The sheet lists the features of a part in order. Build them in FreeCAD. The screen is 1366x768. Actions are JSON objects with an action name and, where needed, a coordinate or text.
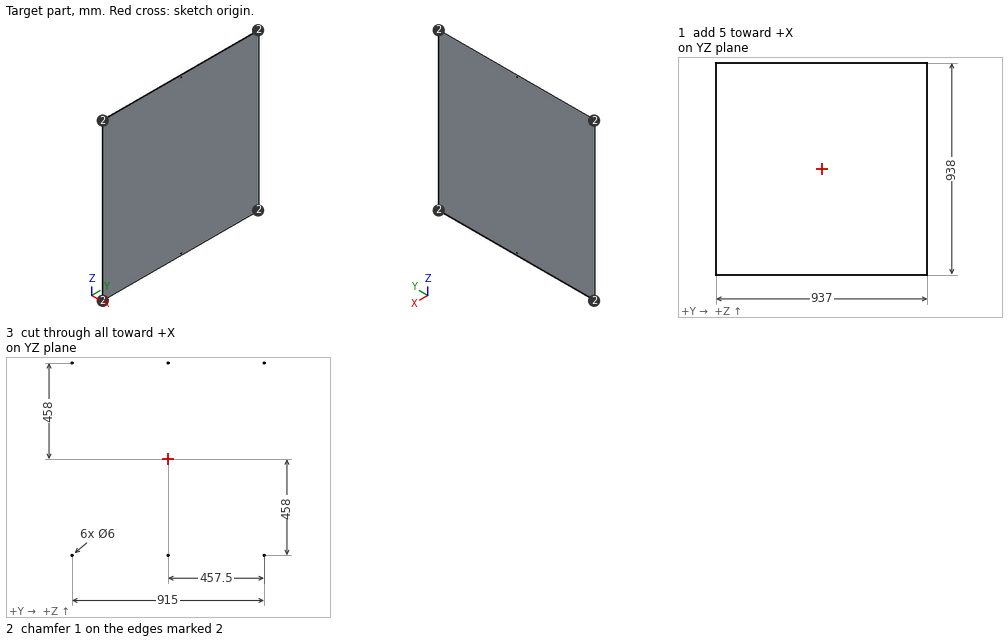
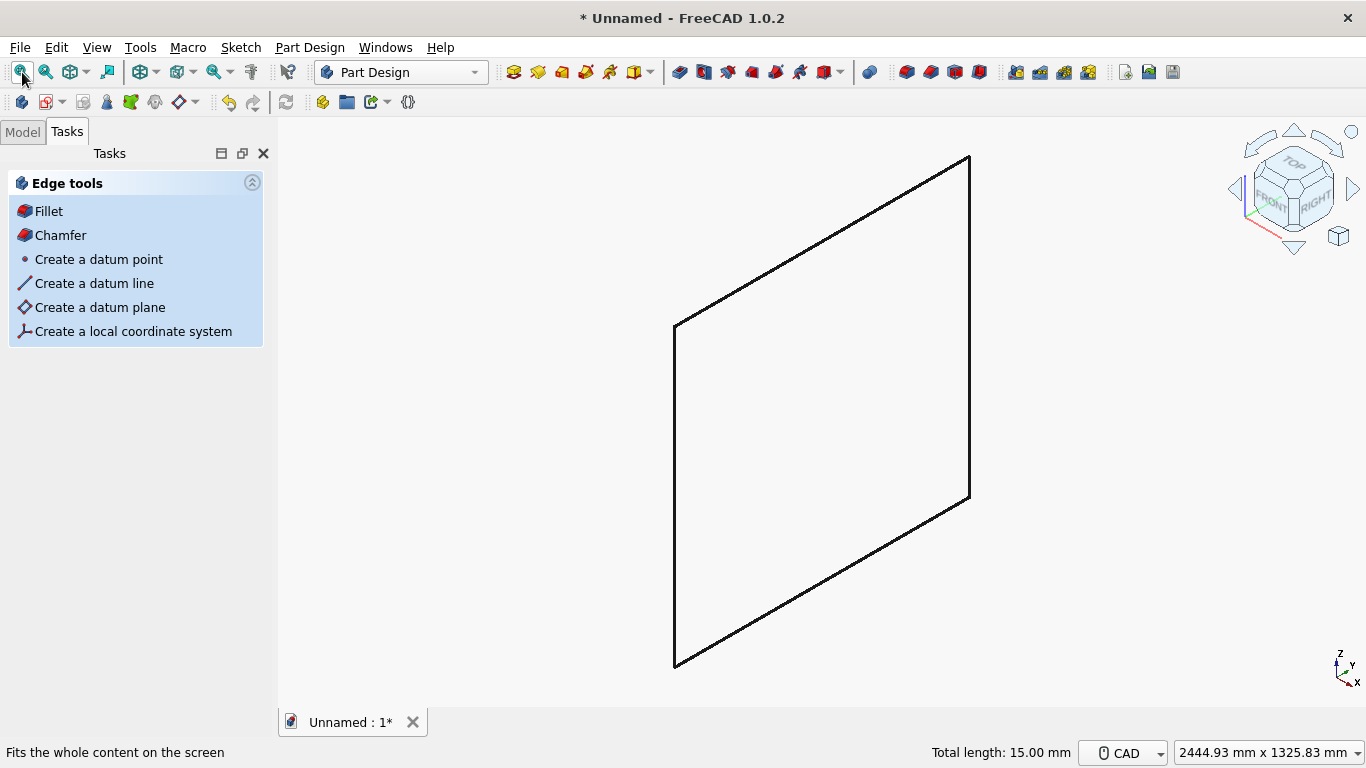
{"action": "scroll", "coordinate": [675, 326], "scroll_direction": "up", "scroll_amount": 15}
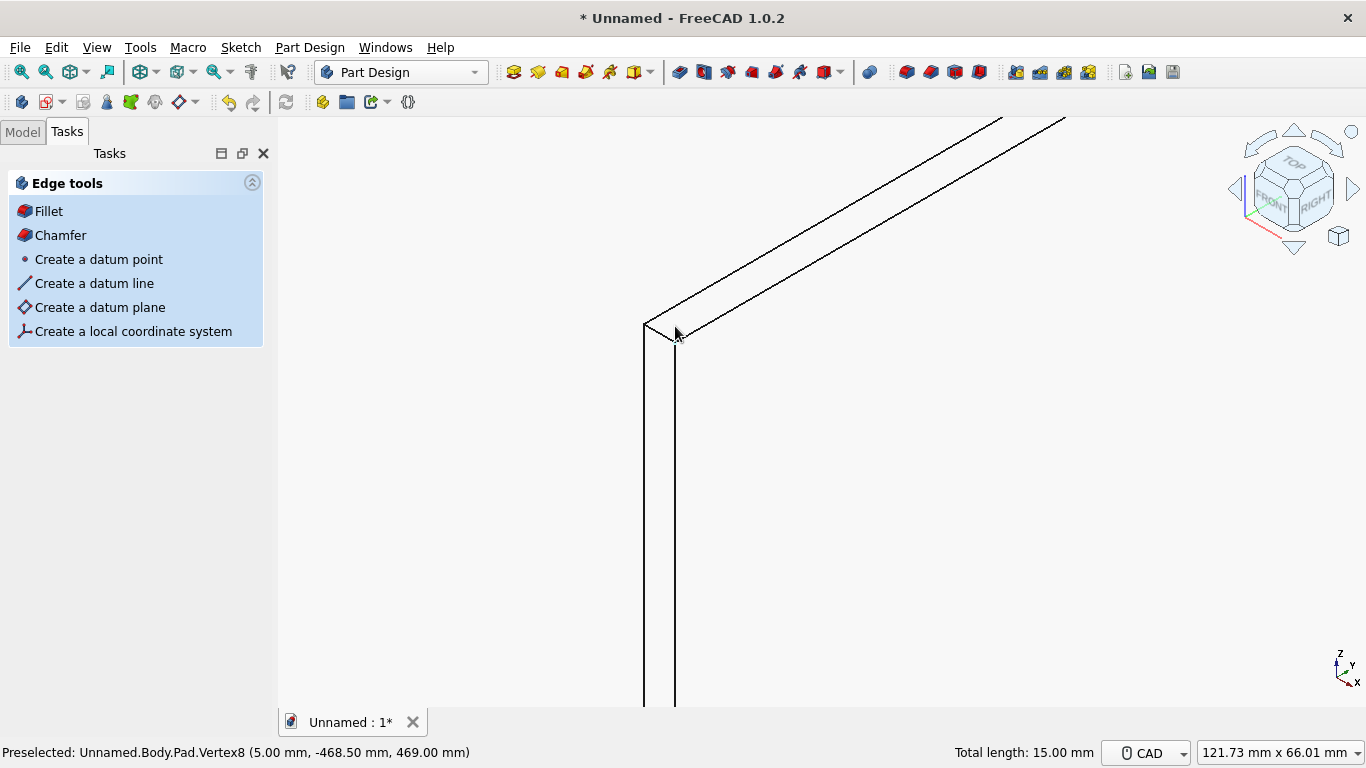
{"action": "left_click", "coordinate": [660, 332], "text": "ctrl"}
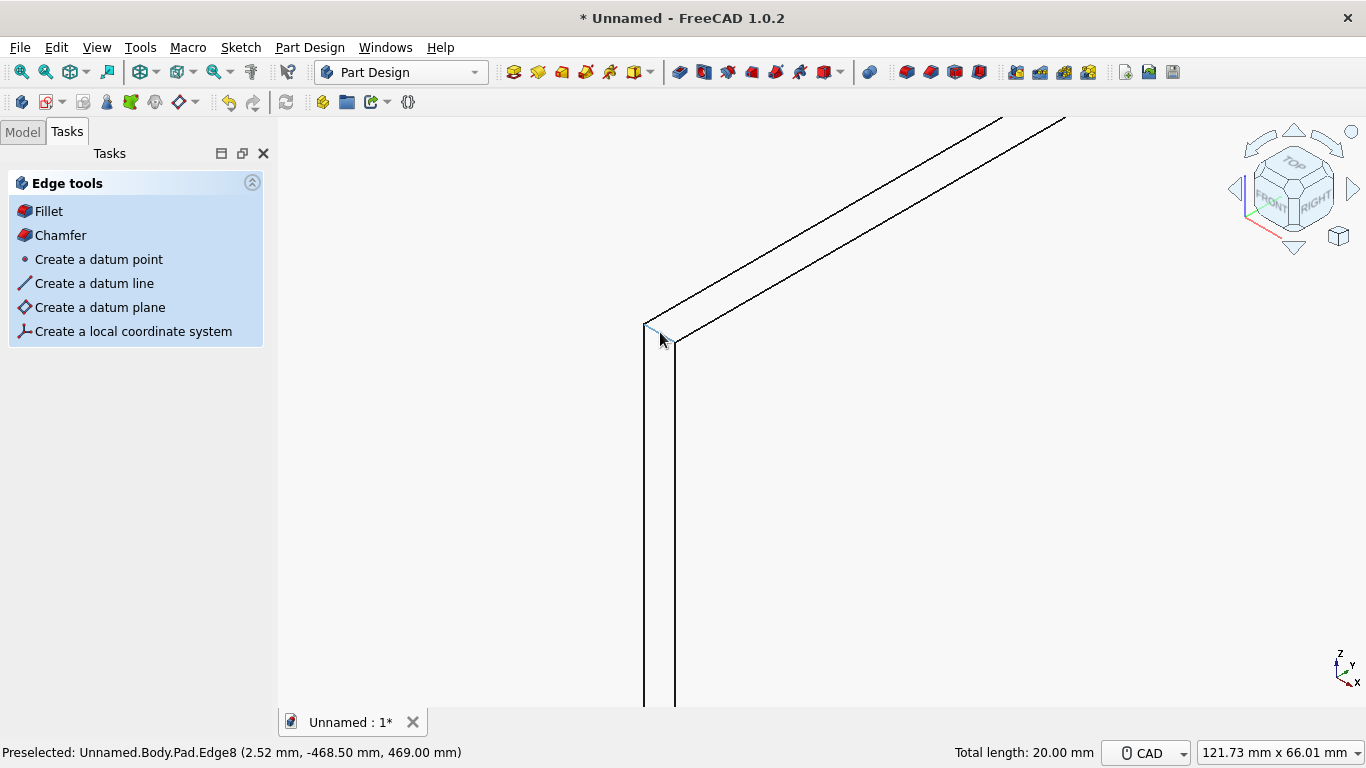
{"action": "key", "text": "v 1"}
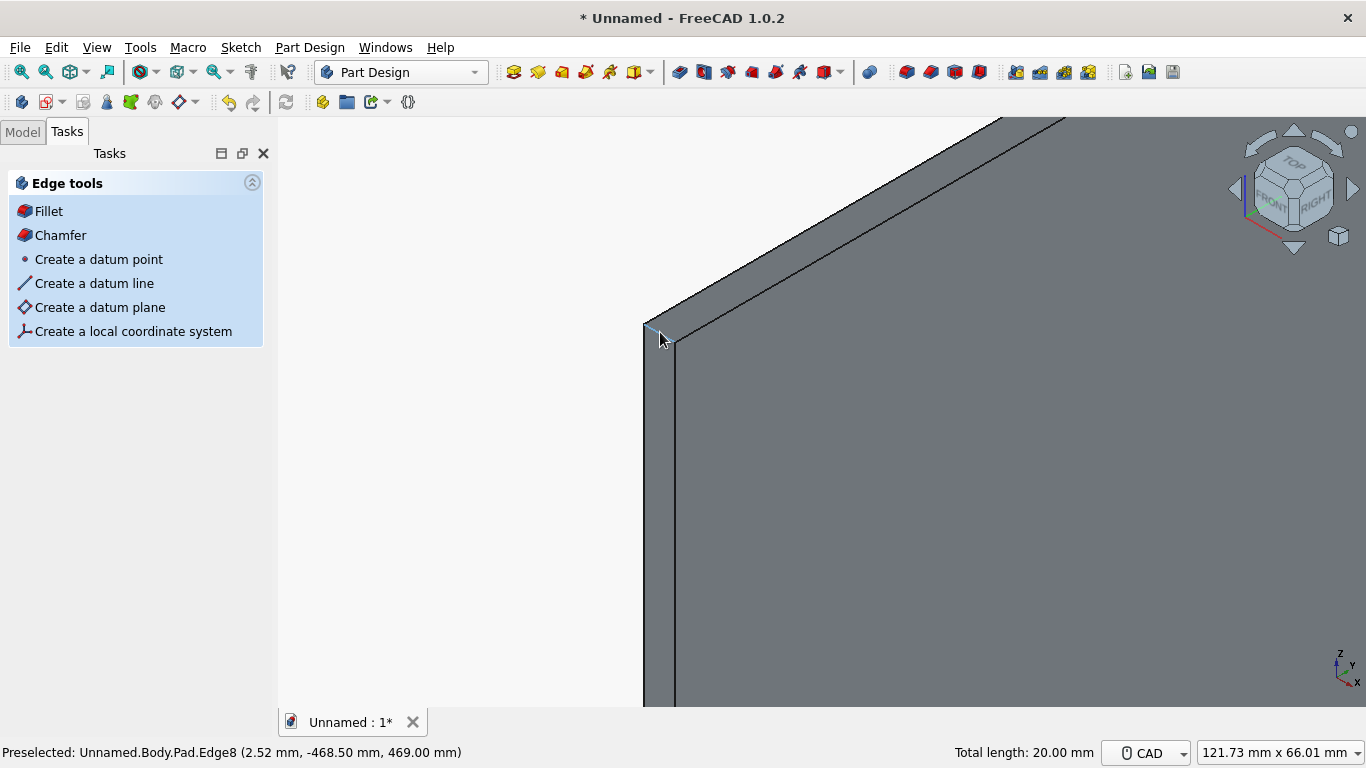
{"action": "left_click", "coordinate": [932, 72]}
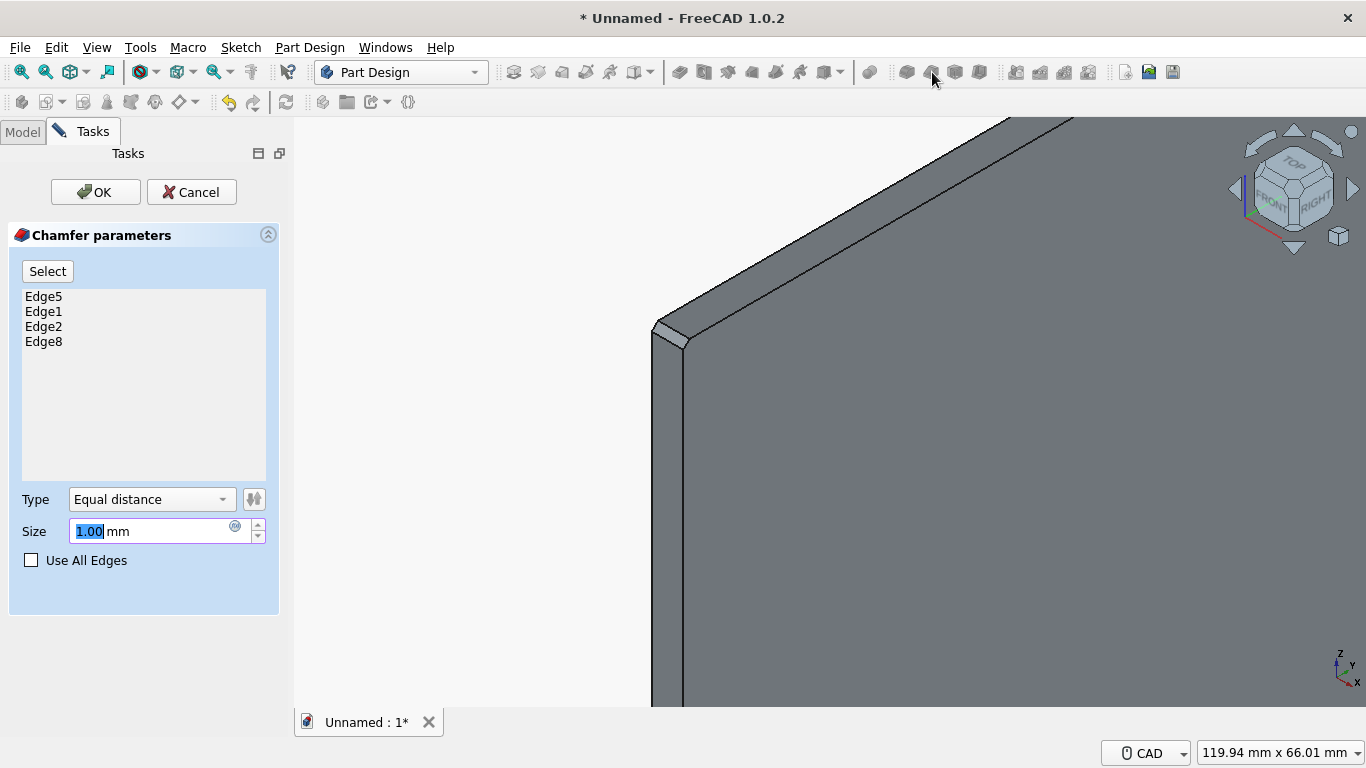
{"action": "type", "text": "1"}
{"action": "key", "text": "Tab"}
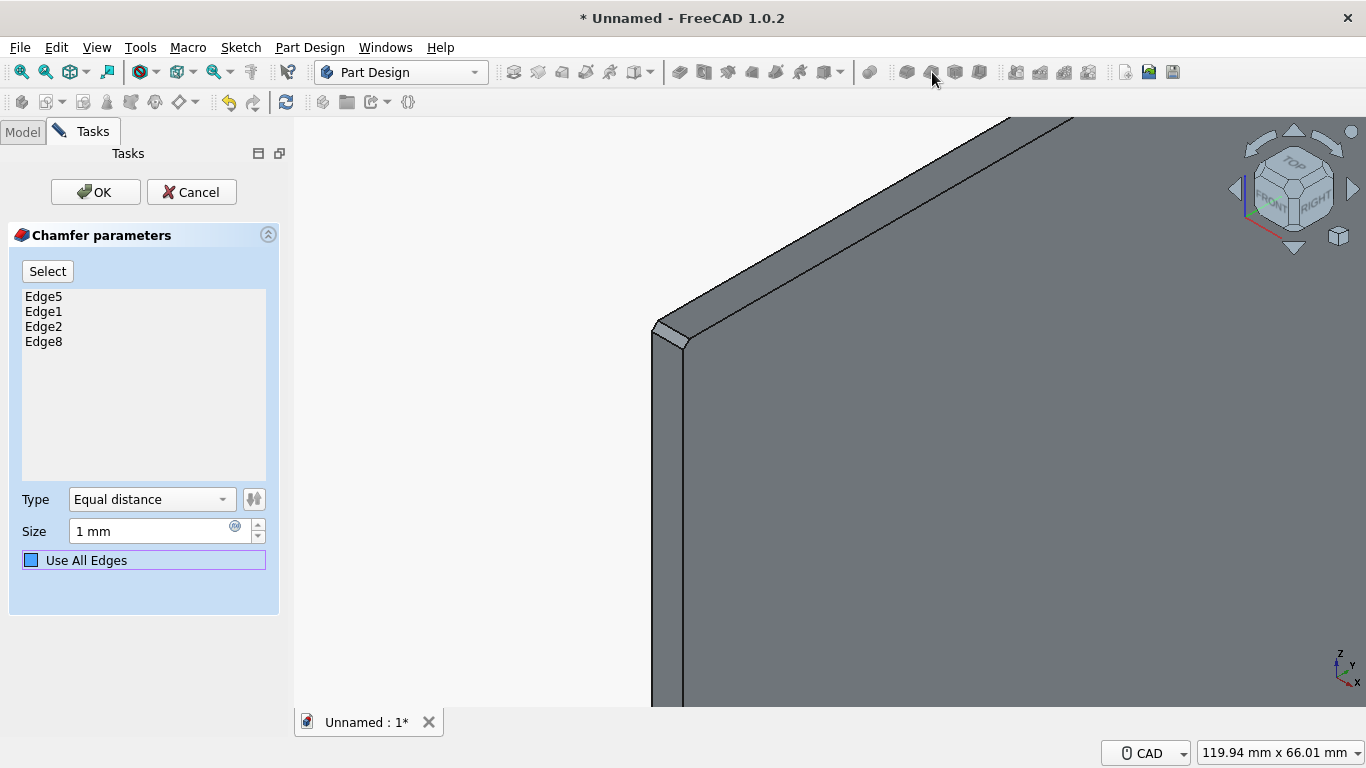
{"action": "left_click", "coordinate": [96, 192]}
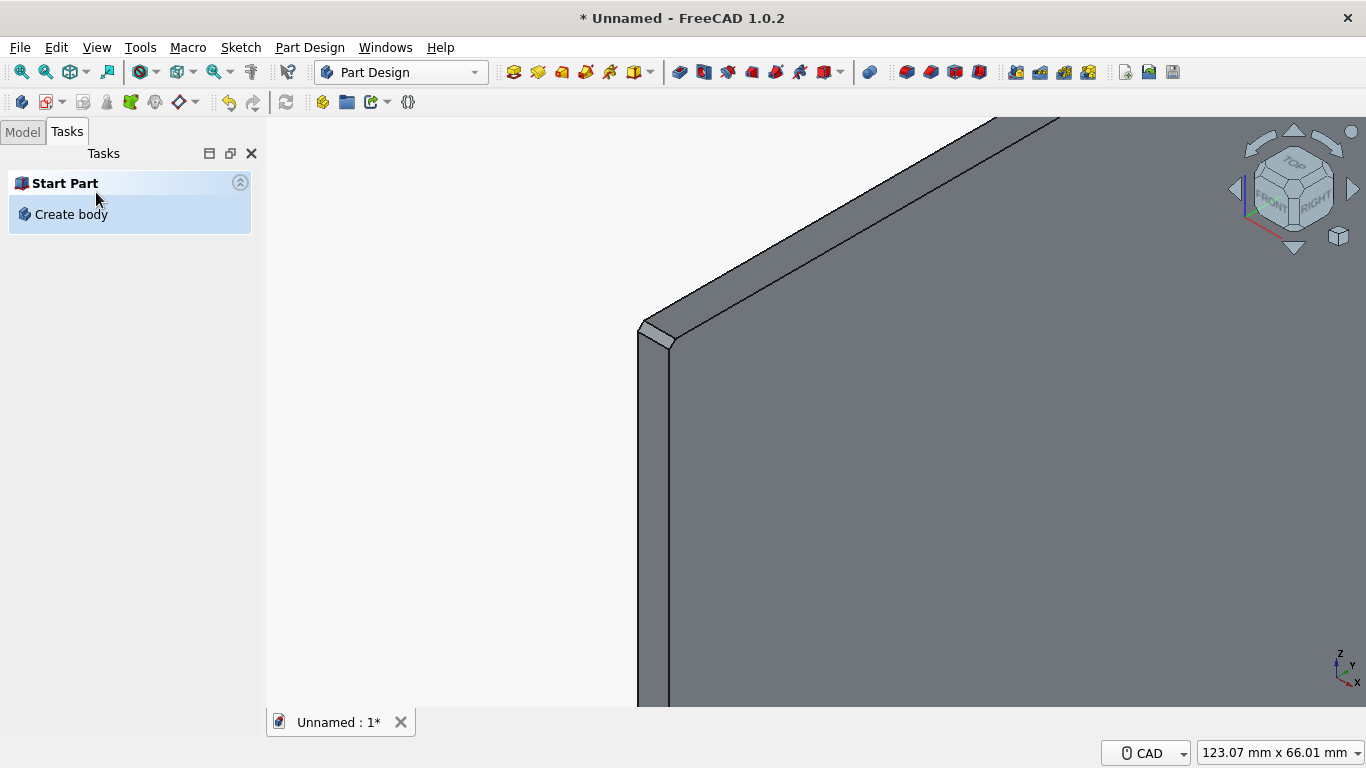
{"action": "left_click", "coordinate": [22, 72]}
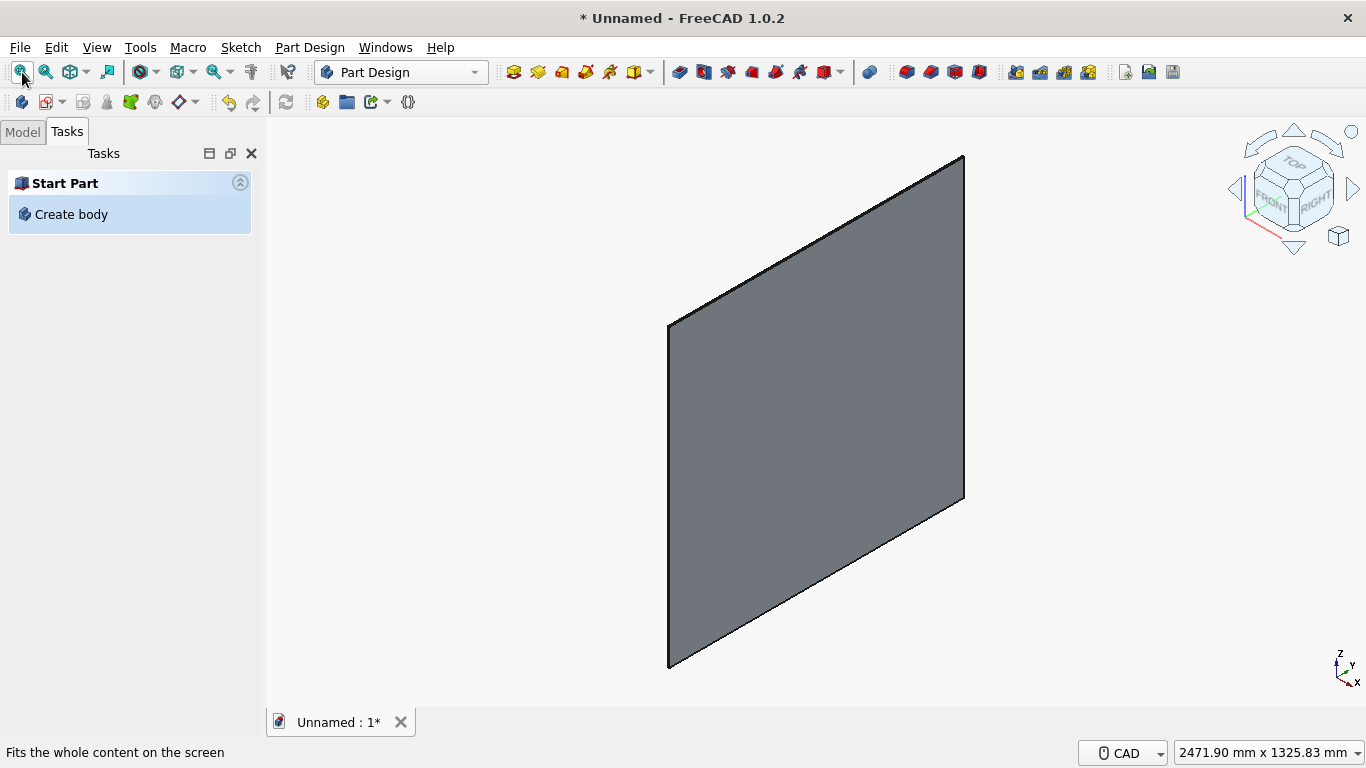
{"action": "left_click", "coordinate": [46, 102]}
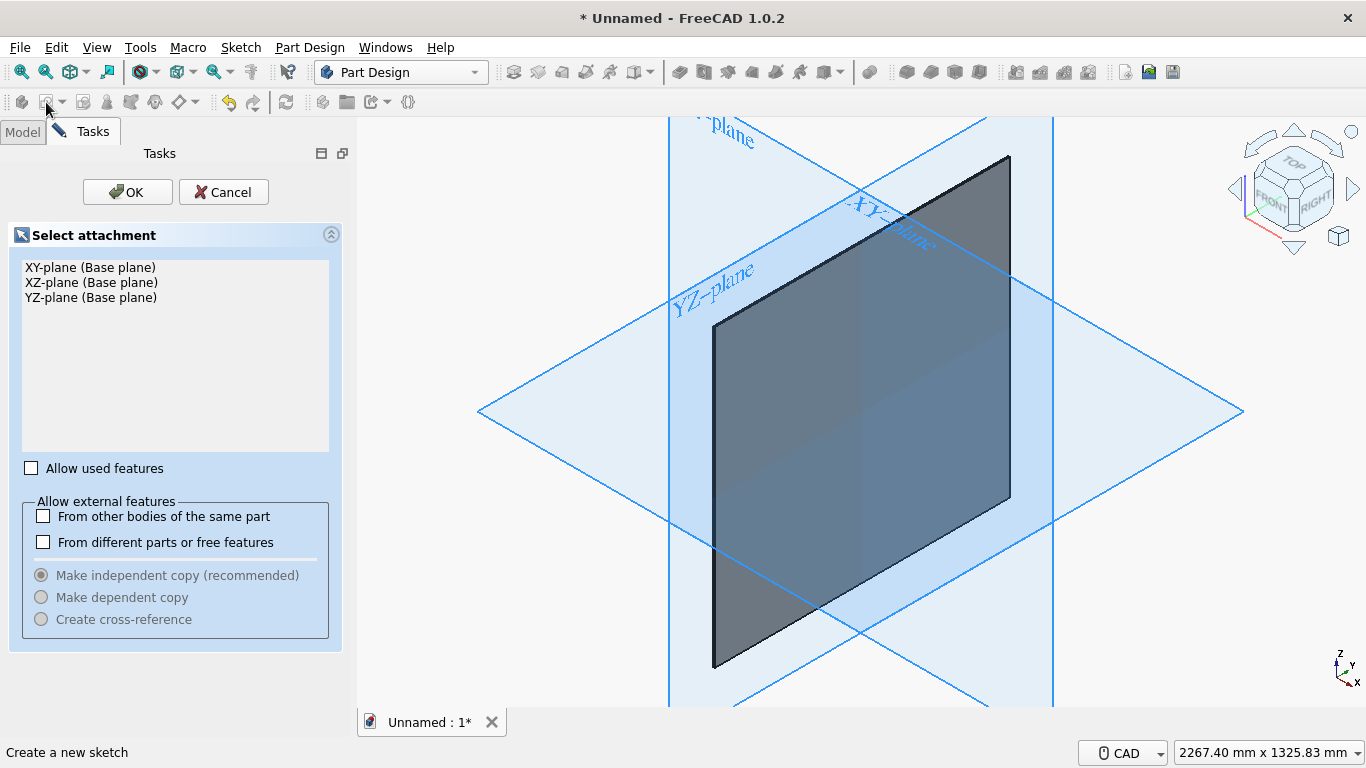
{"action": "left_click", "coordinate": [82, 298]}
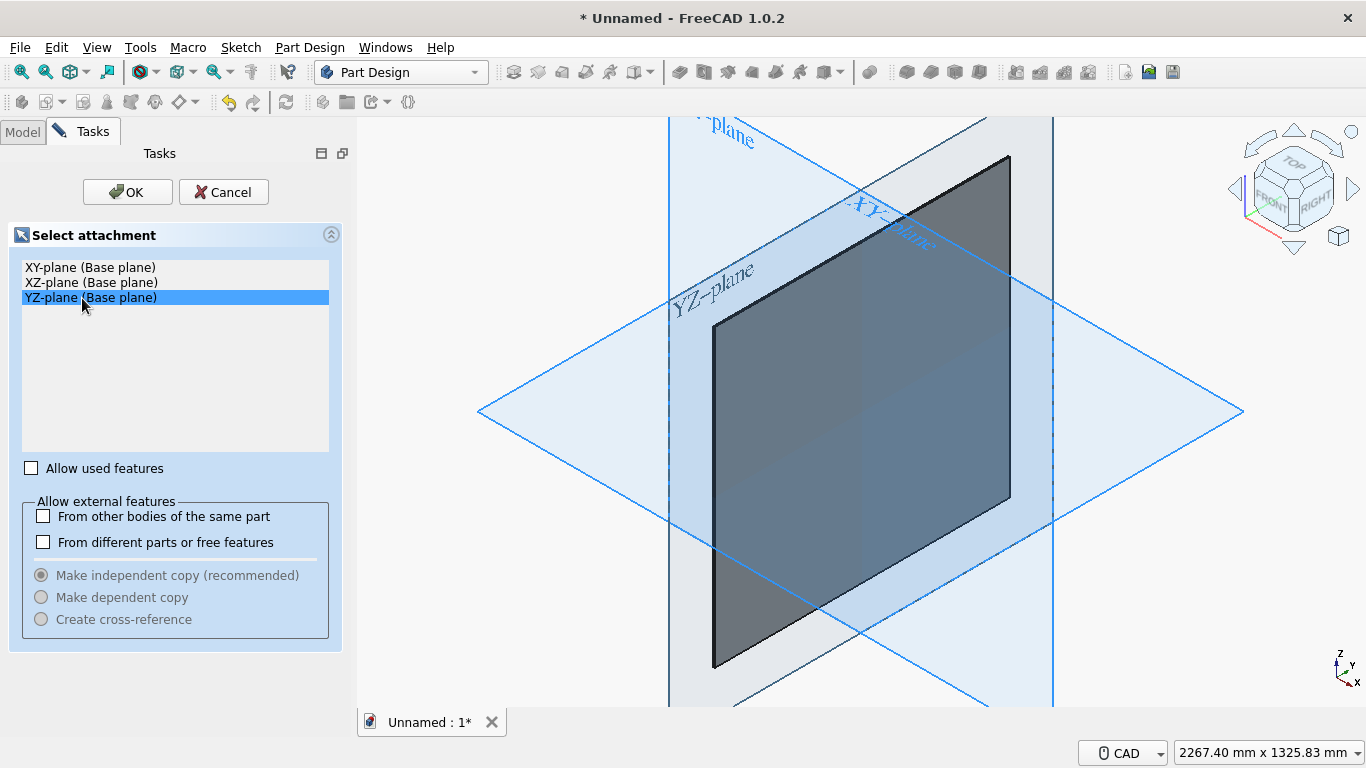
{"action": "left_click", "coordinate": [128, 192]}